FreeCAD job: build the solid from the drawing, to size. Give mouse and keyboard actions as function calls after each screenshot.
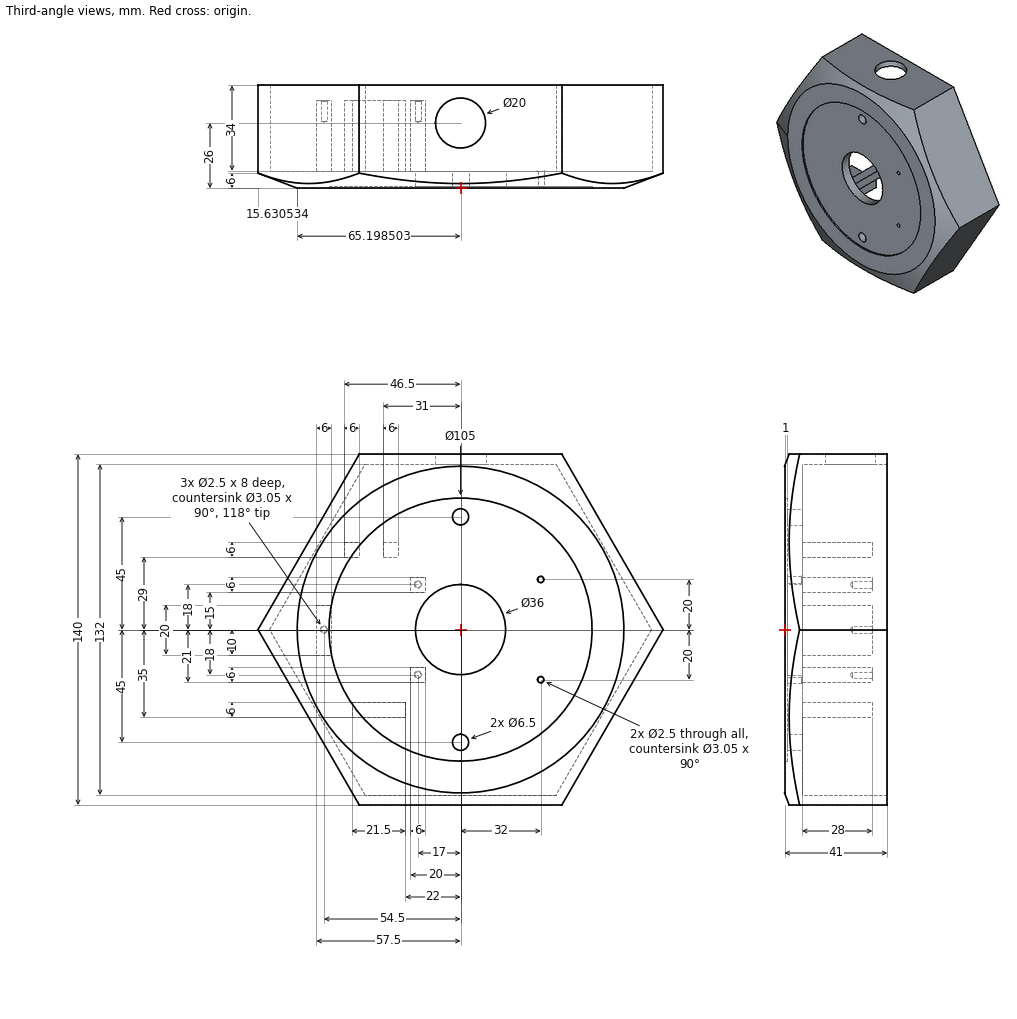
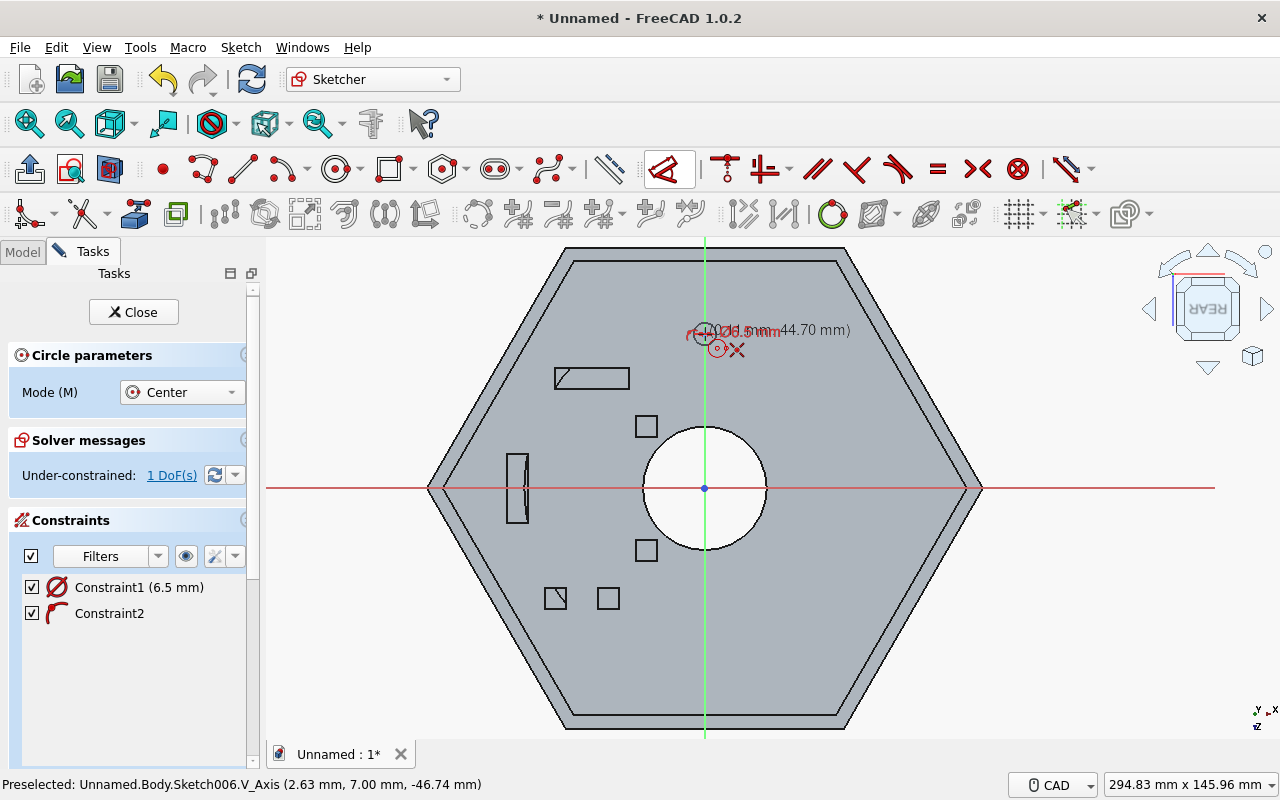
scroll(705, 643, up, 4)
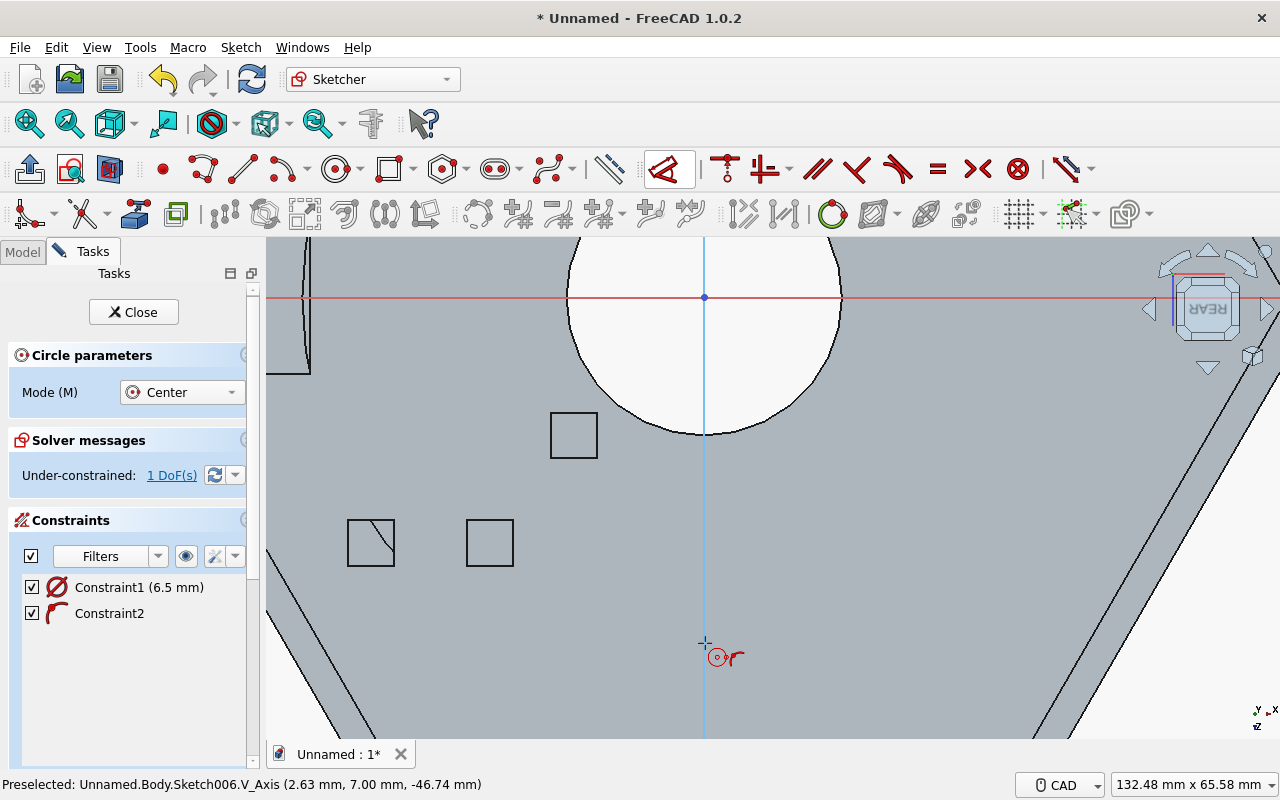
click(704, 642)
move(722, 625)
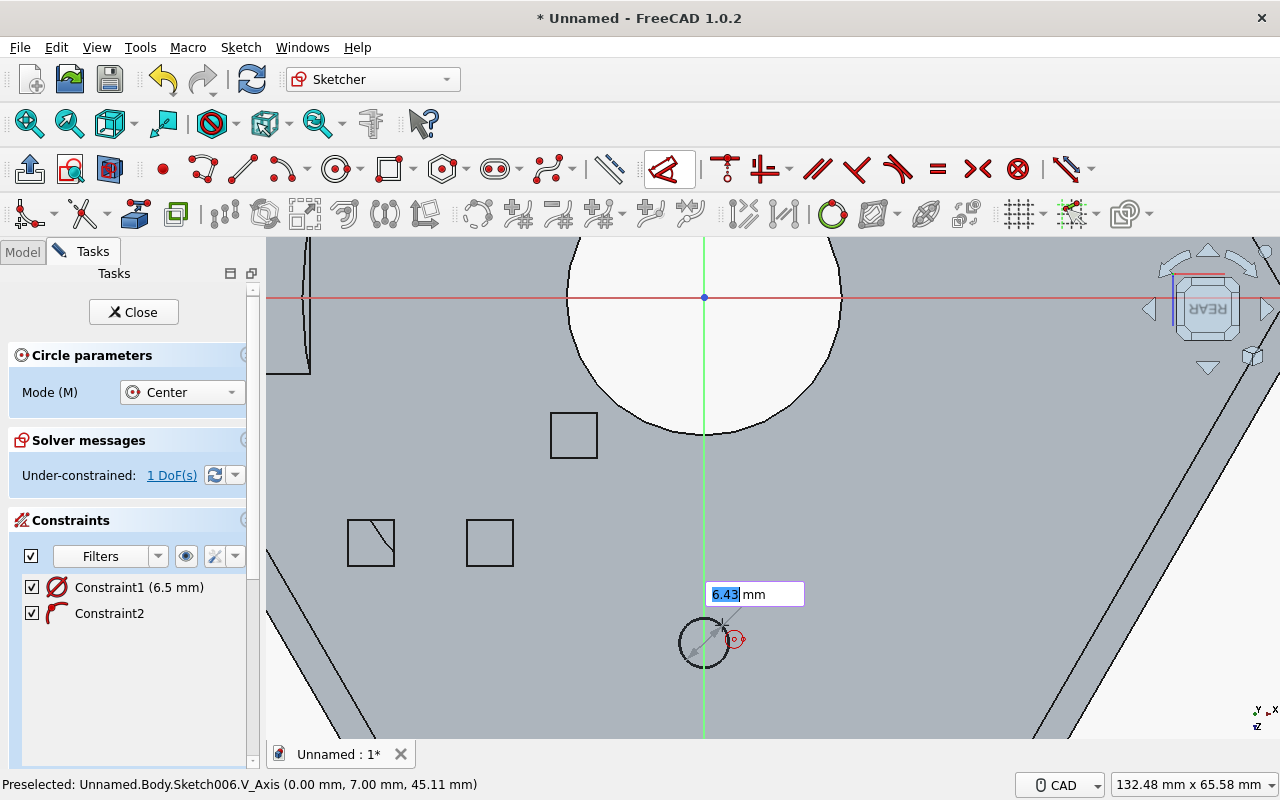
text(6.5)
key(Return)
key(Escape)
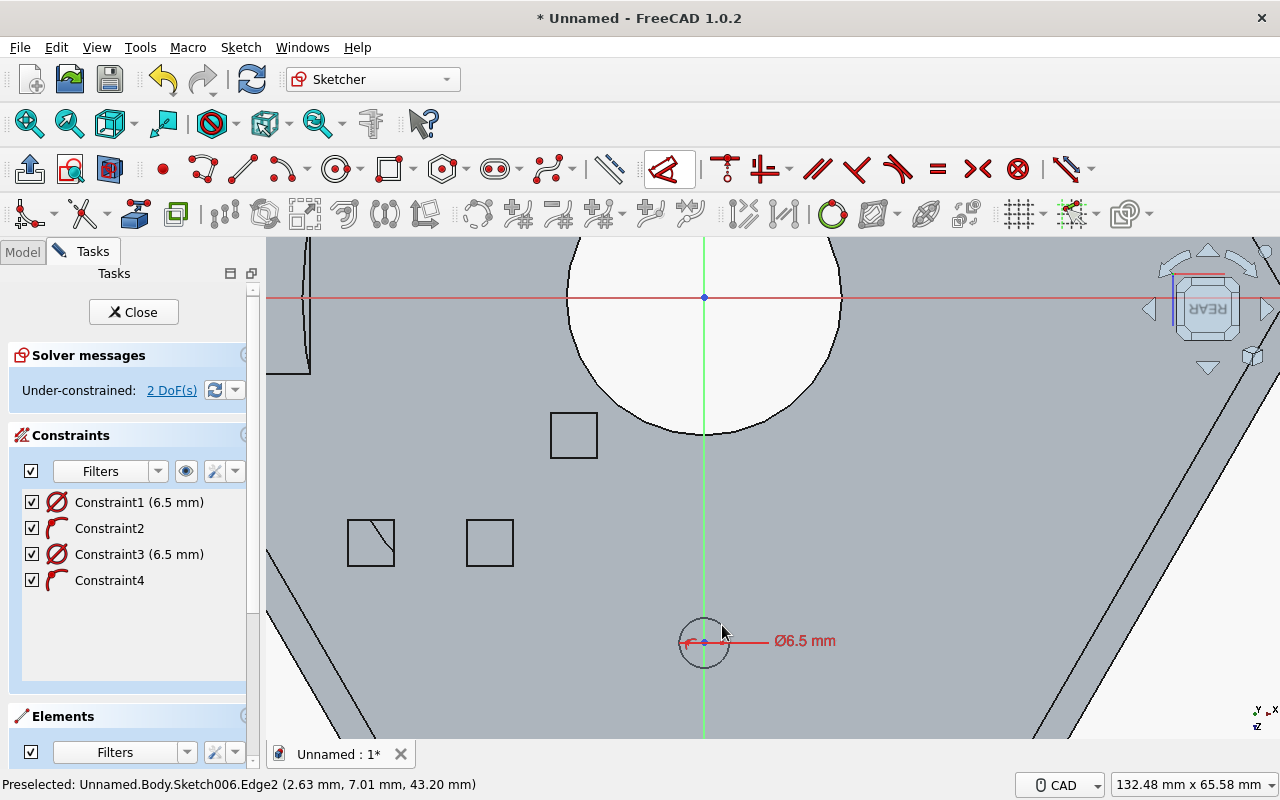
scroll(705, 643, down, 4)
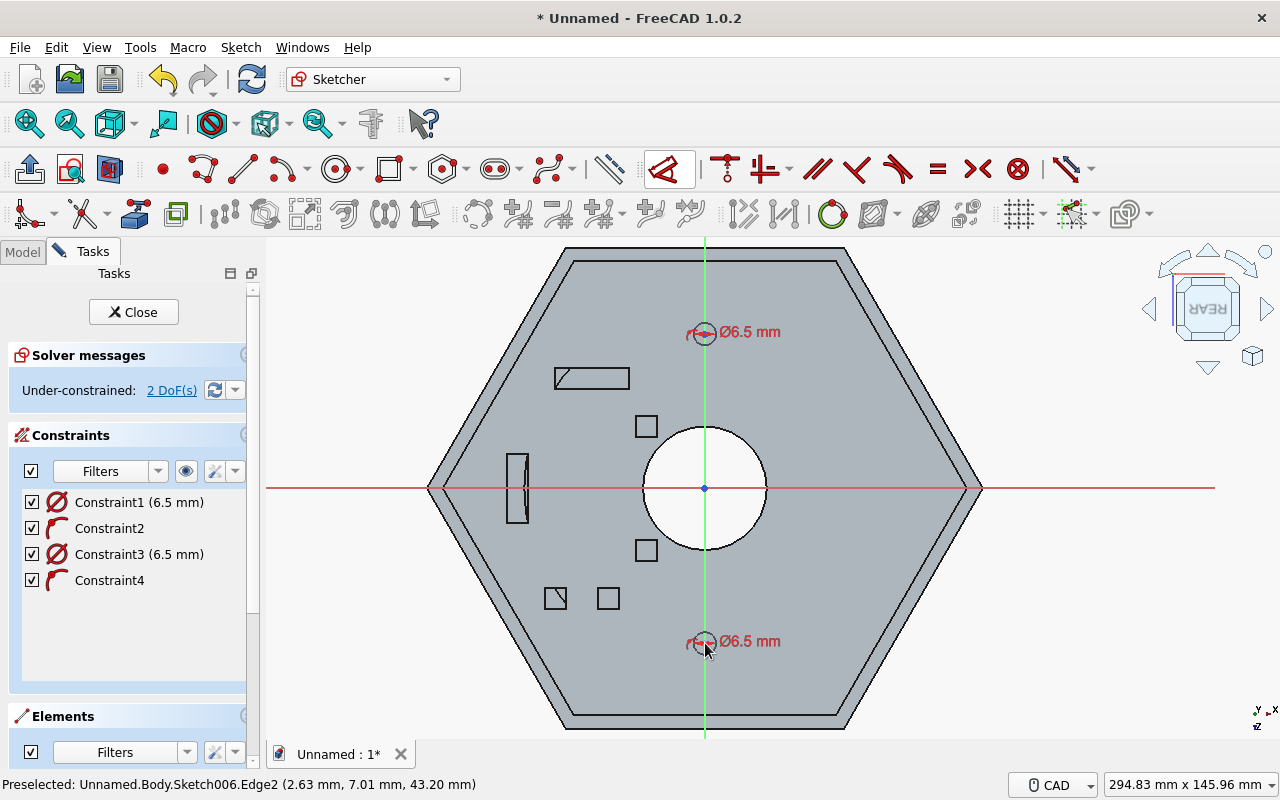
click(705, 334)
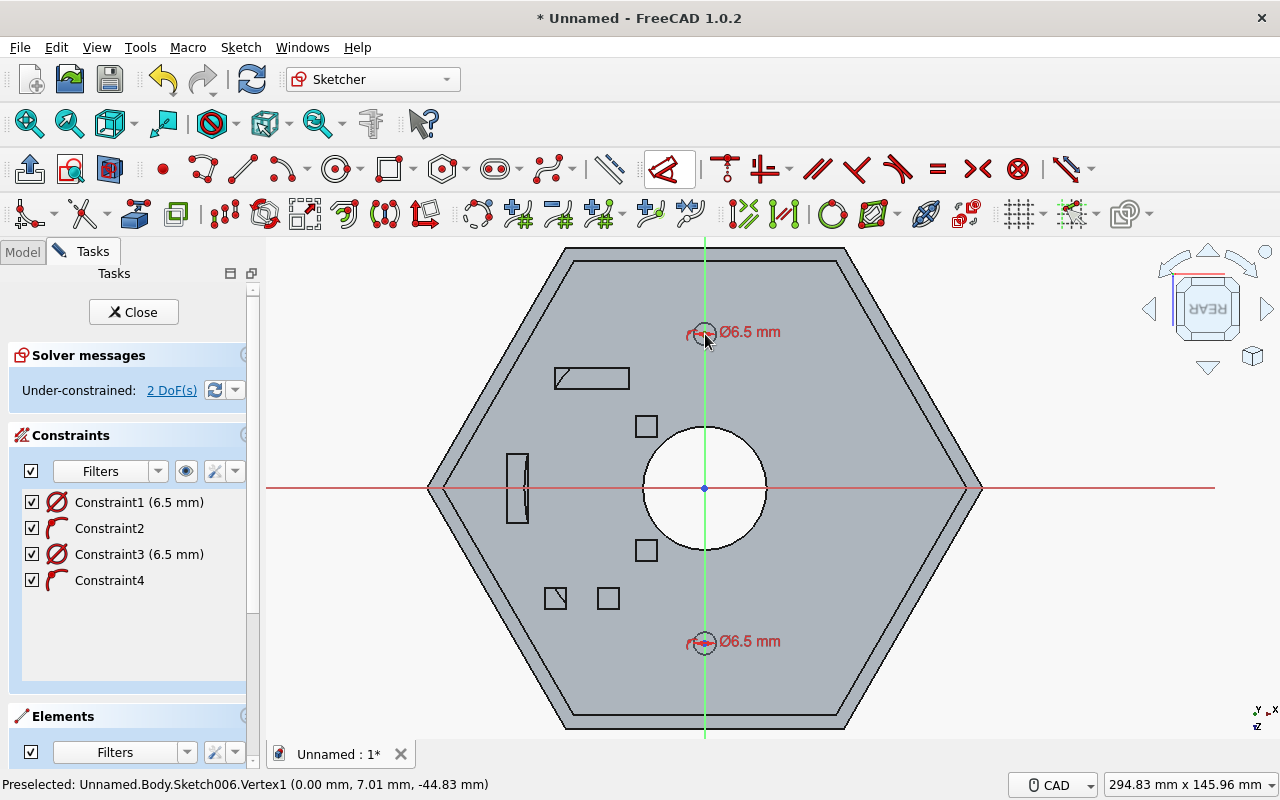
click(690, 170)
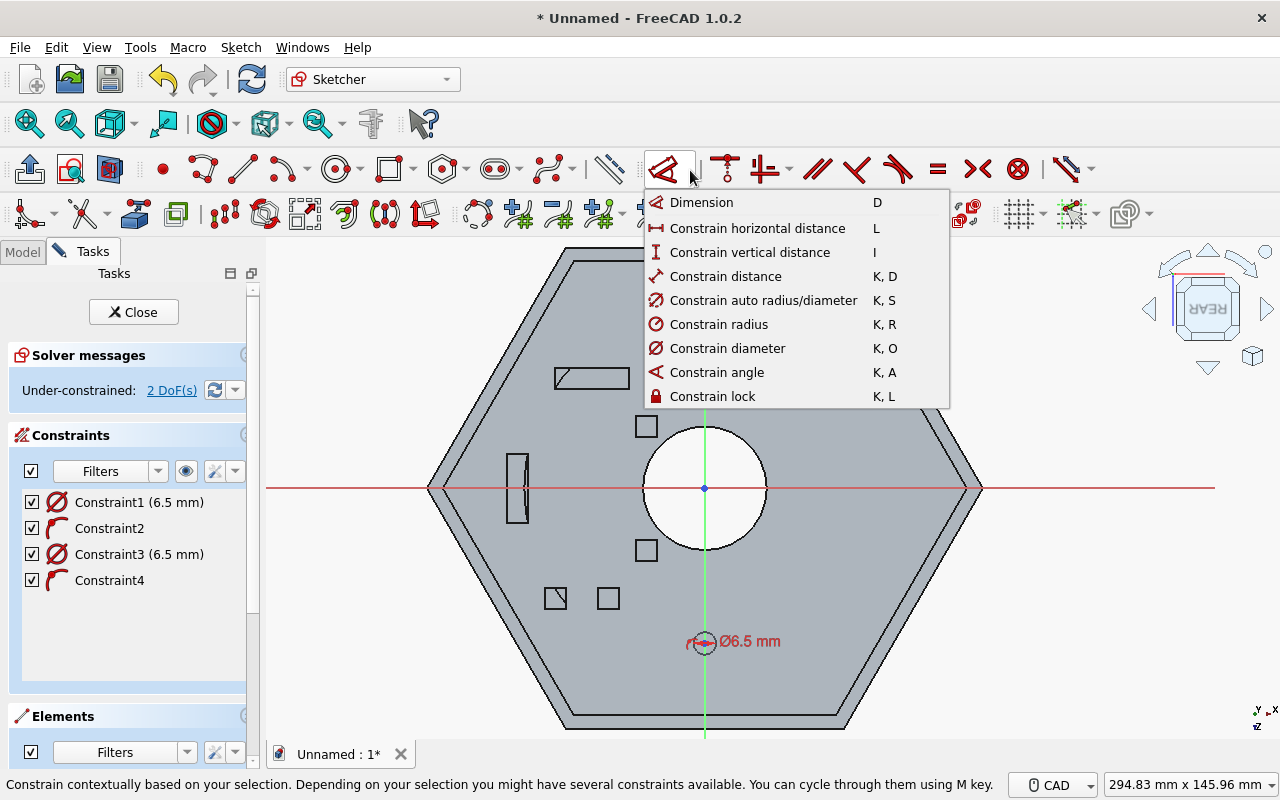
click(797, 252)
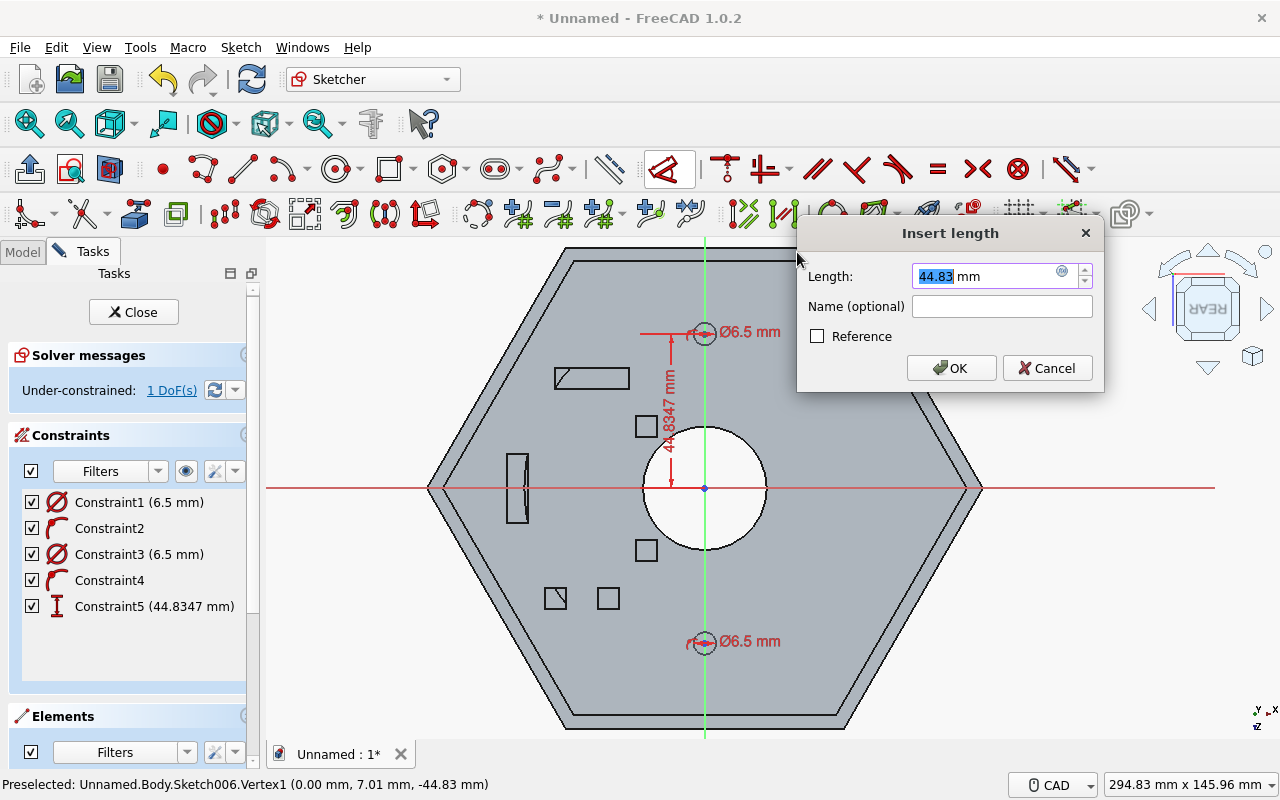
text(45)
key(Return)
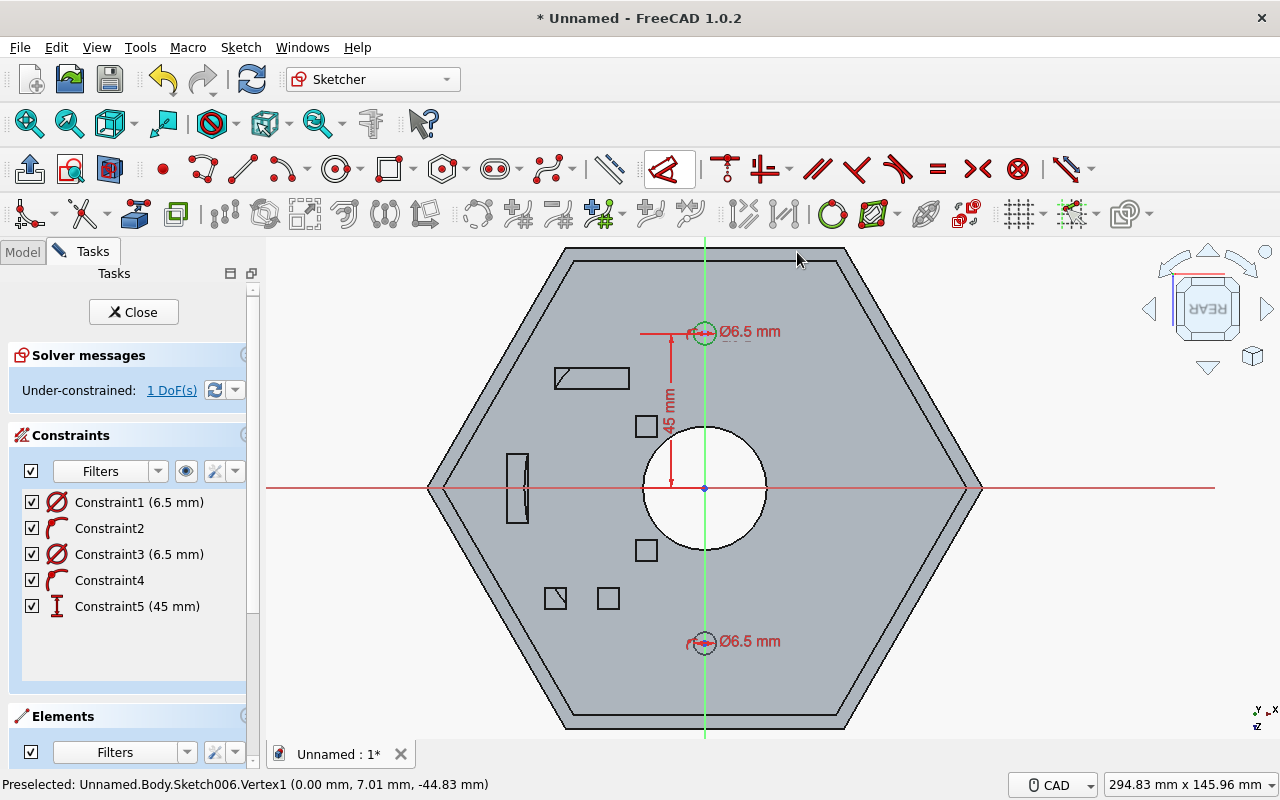
click(705, 643)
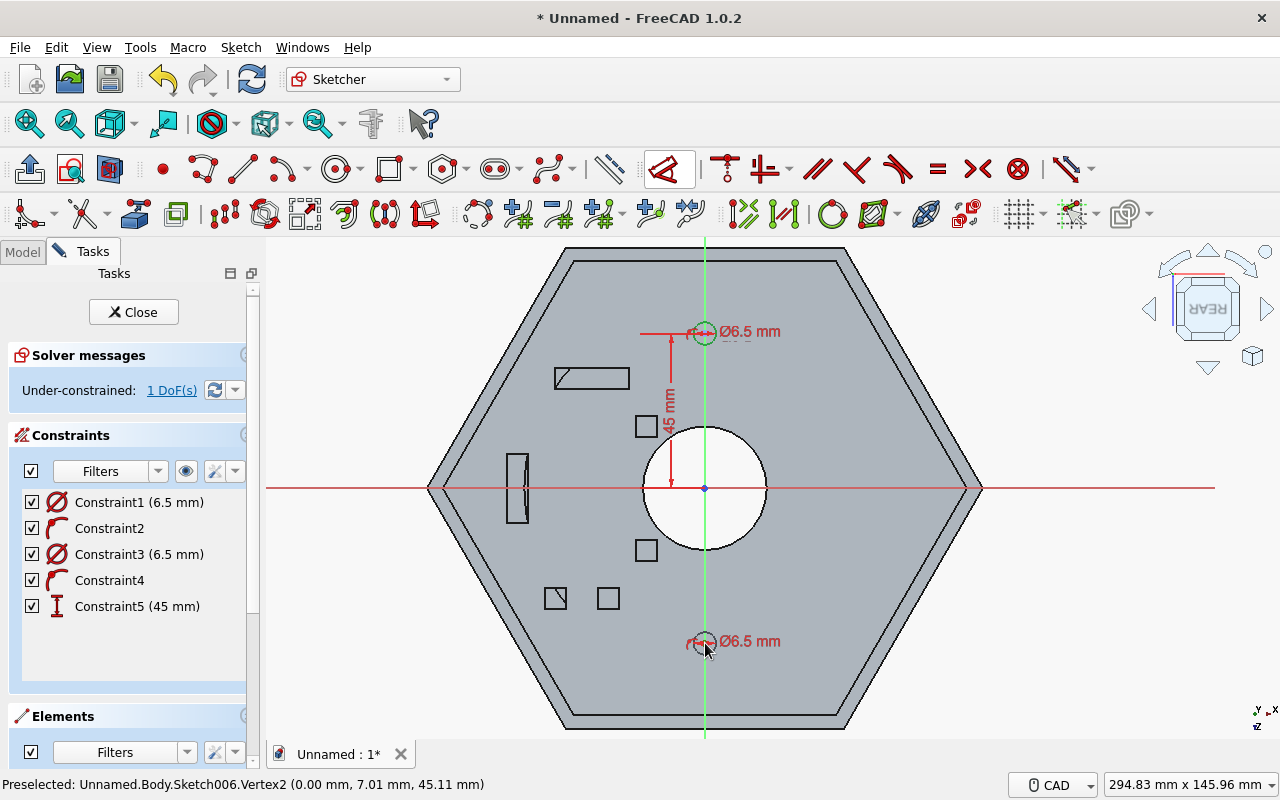
key(i)